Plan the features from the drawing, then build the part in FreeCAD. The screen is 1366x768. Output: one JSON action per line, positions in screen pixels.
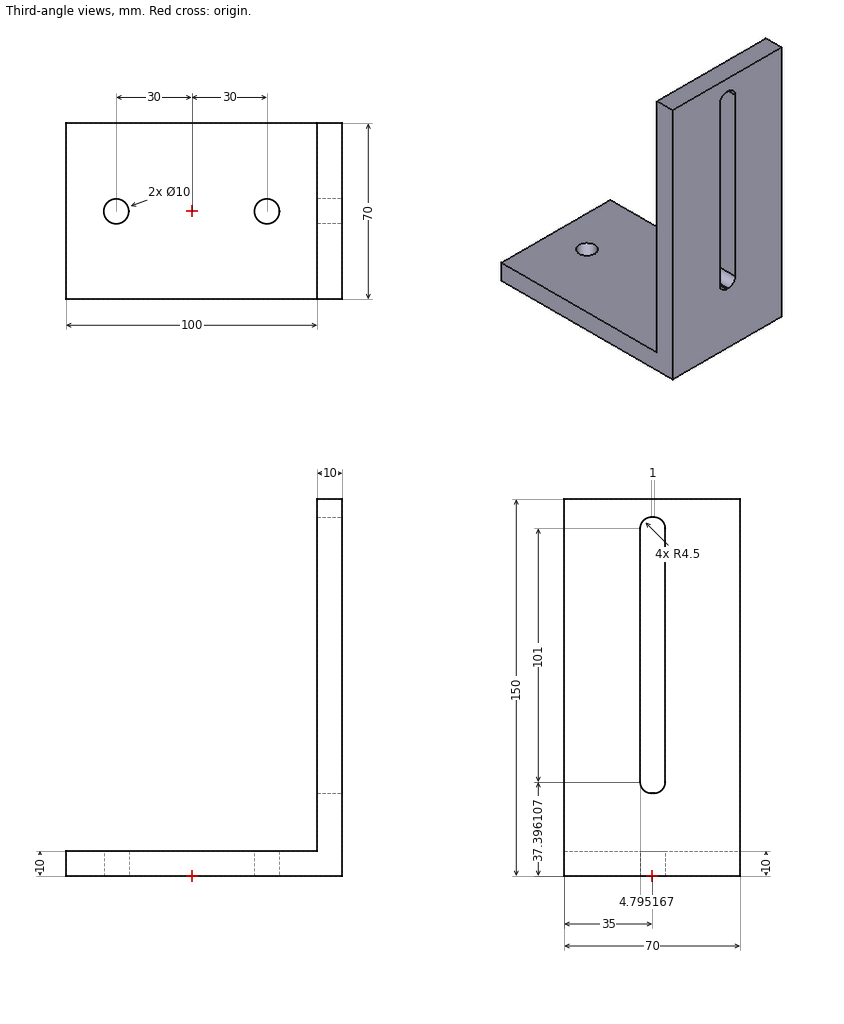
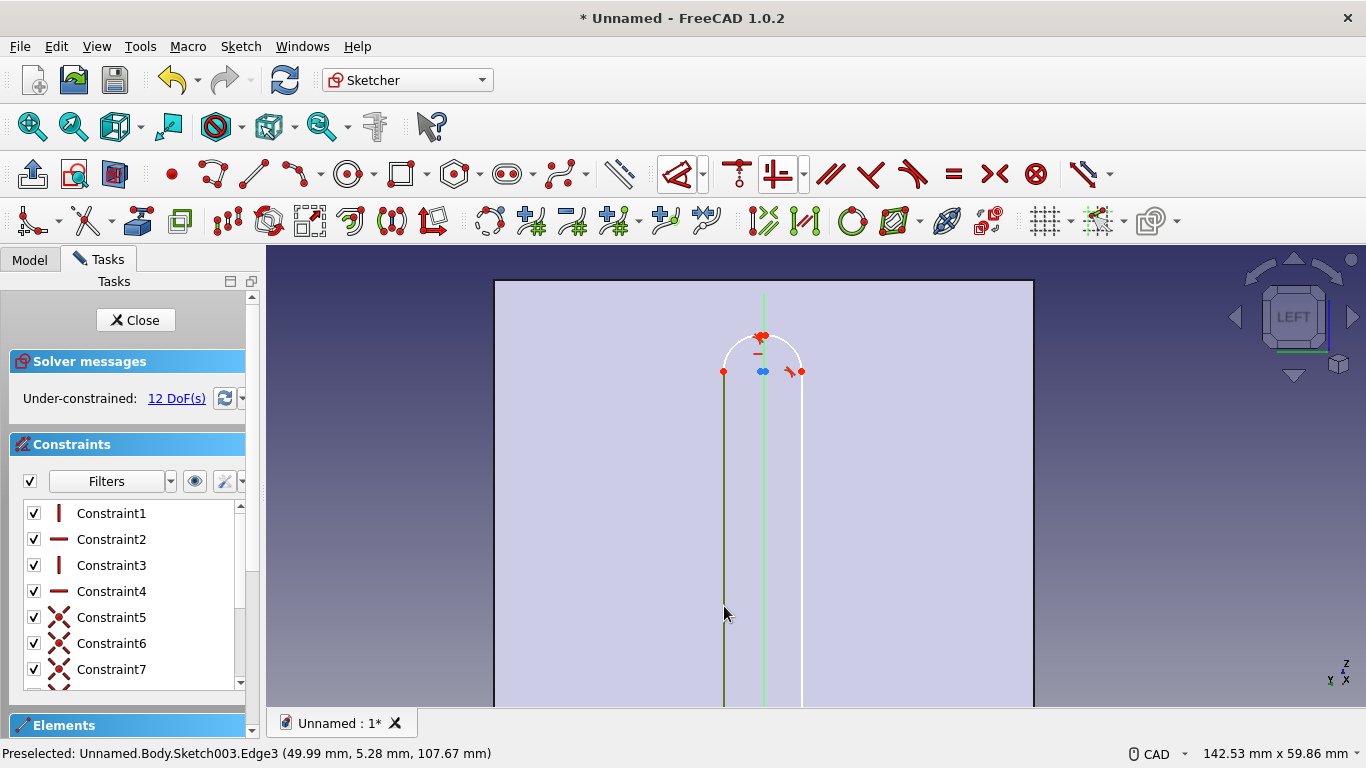
{"action": "left_click", "coordinate": [744, 339]}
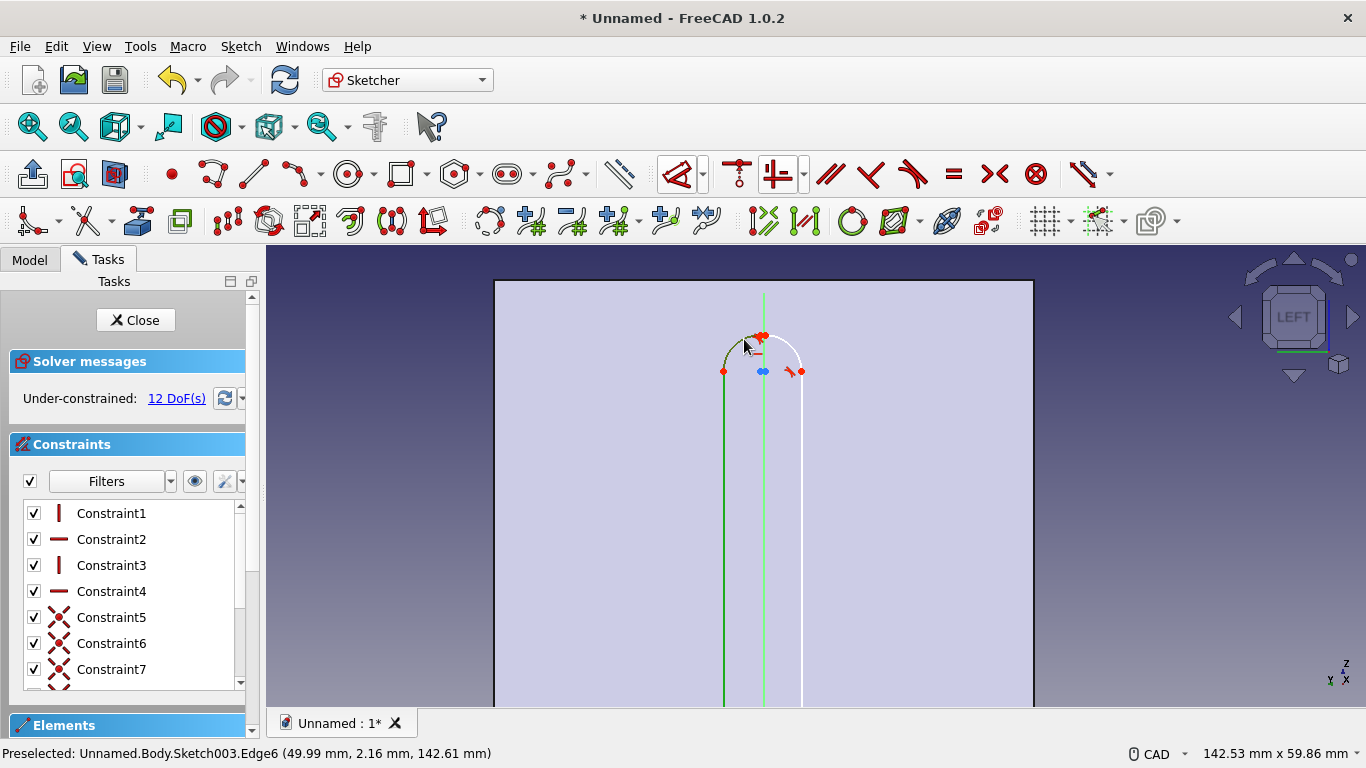
{"action": "left_click", "coordinate": [913, 174]}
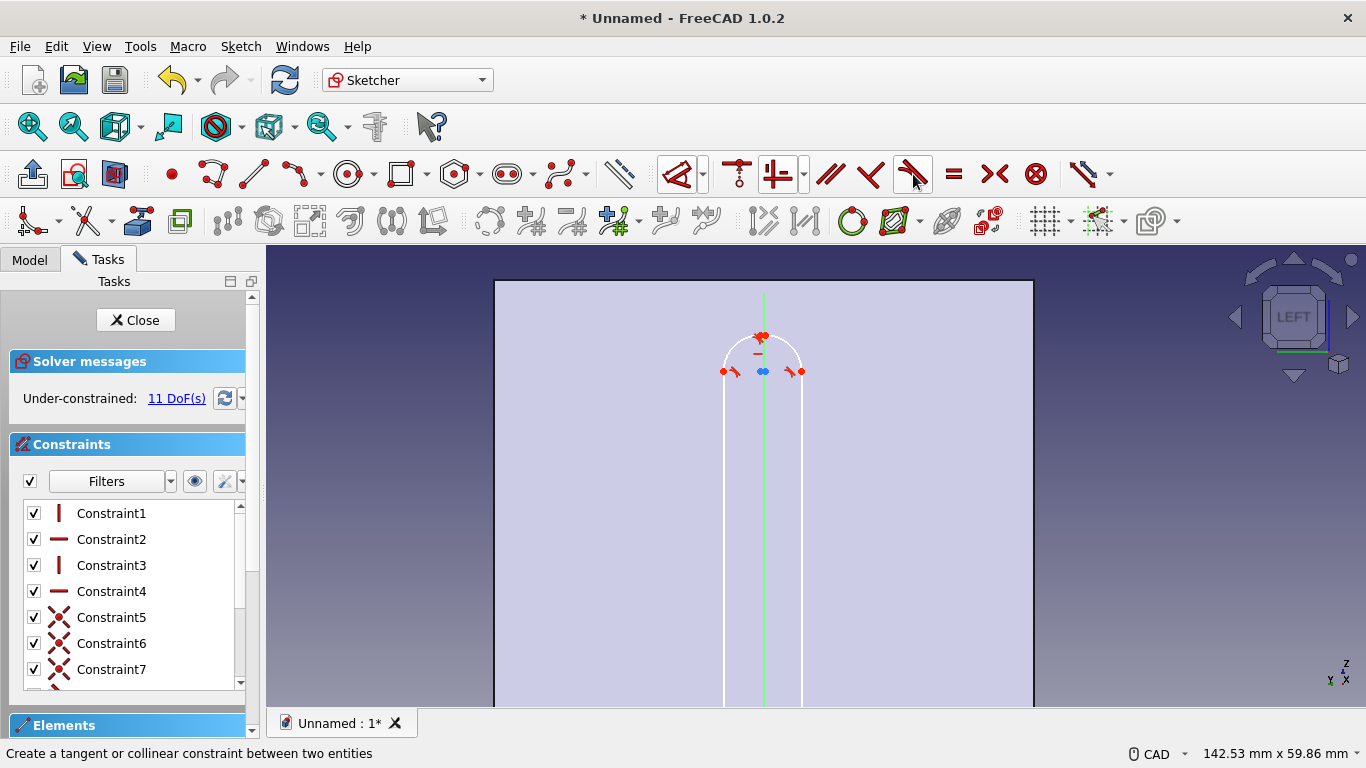
{"action": "left_click", "coordinate": [724, 606]}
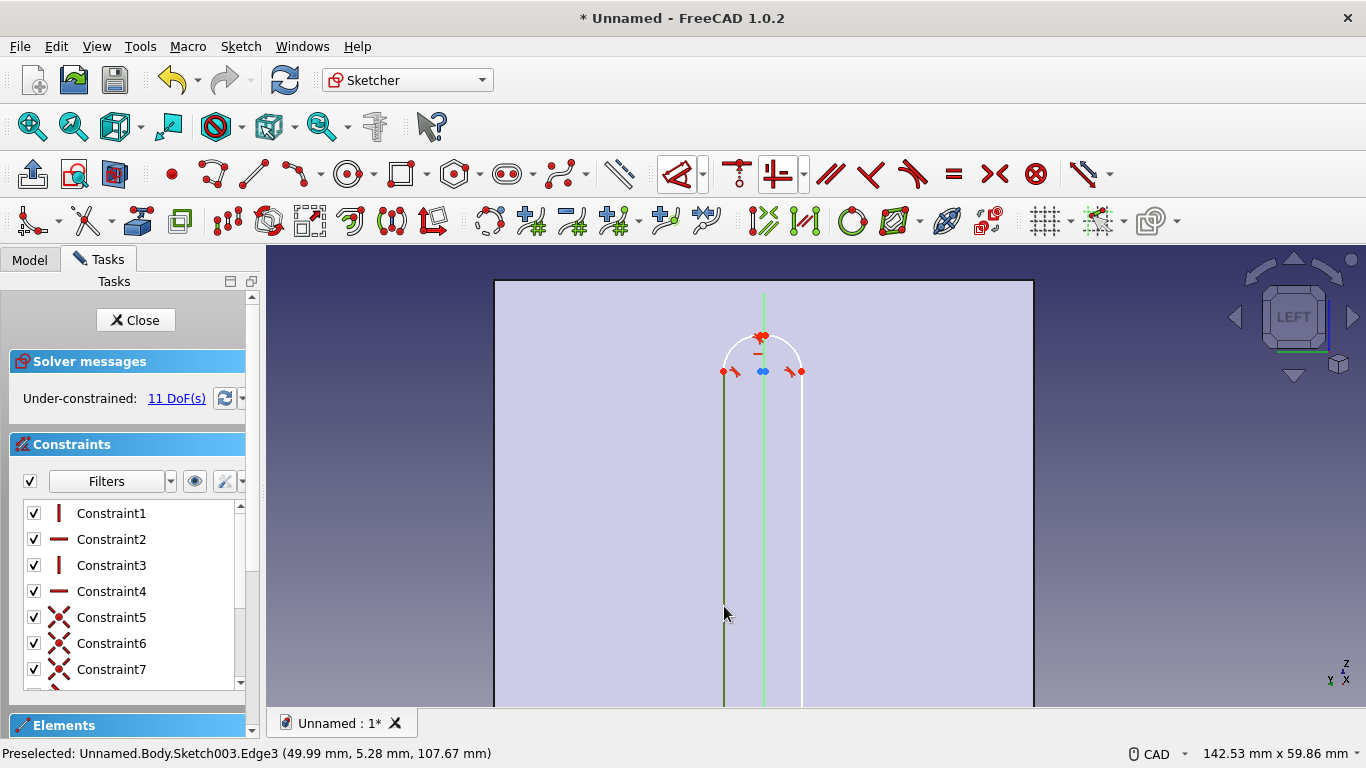
{"action": "scroll", "coordinate": [742, 342], "scroll_direction": "down", "scroll_amount": 7}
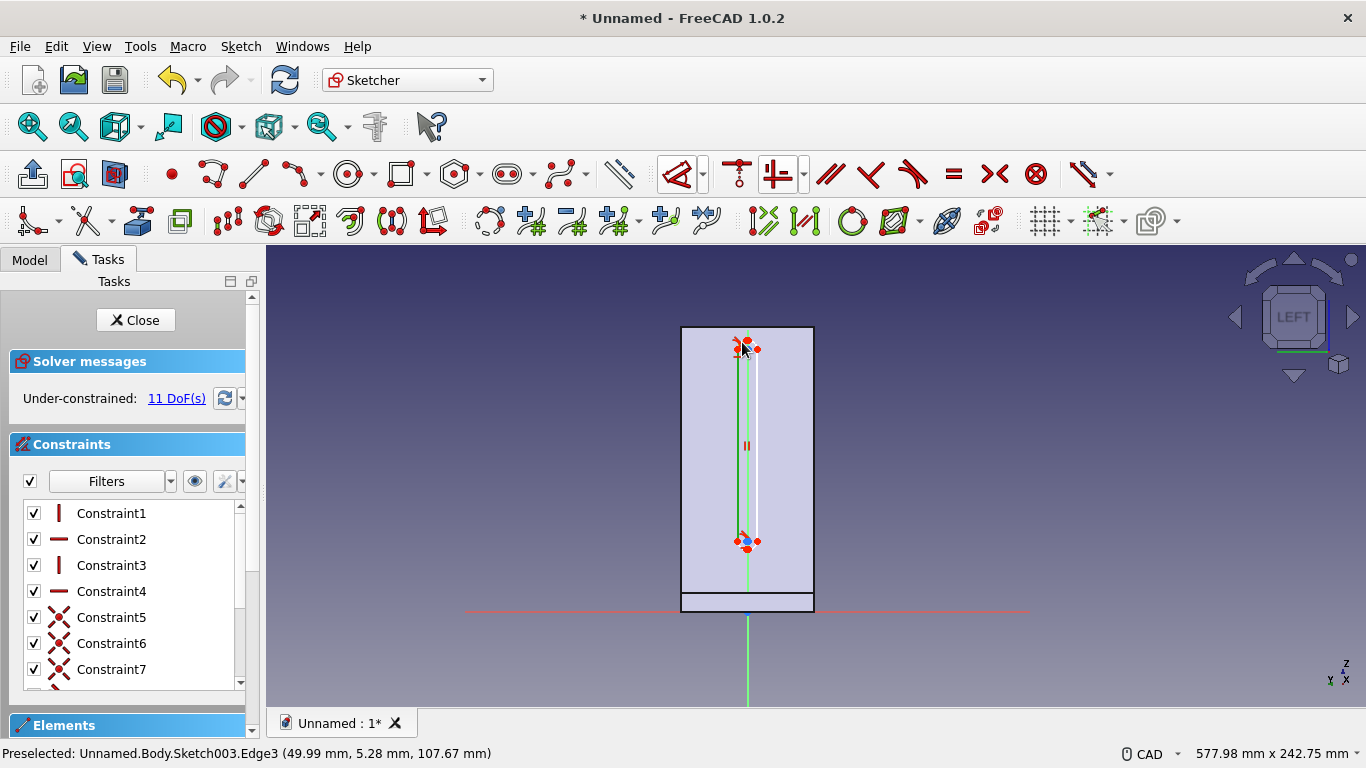
{"action": "scroll", "coordinate": [739, 545], "scroll_direction": "up", "scroll_amount": 7}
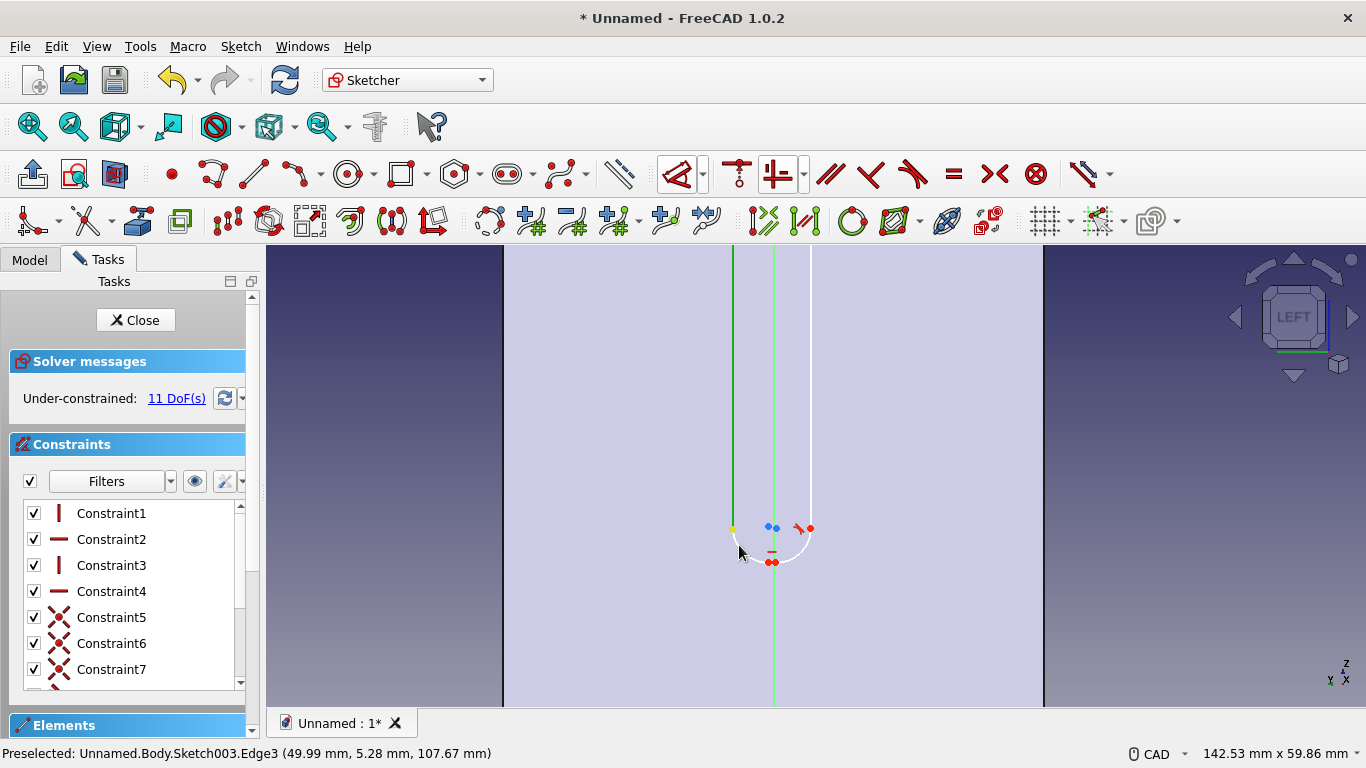
{"action": "left_click", "coordinate": [737, 545]}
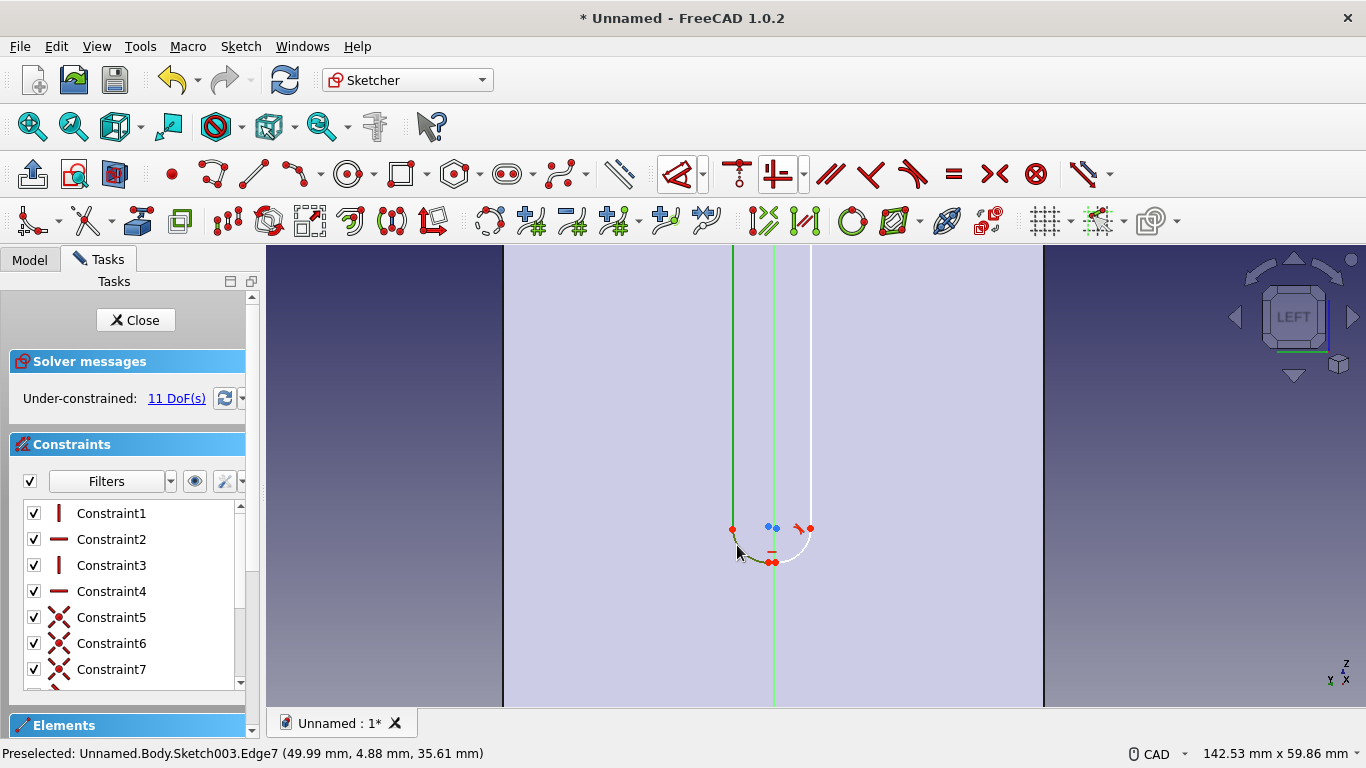
{"action": "left_click", "coordinate": [913, 174]}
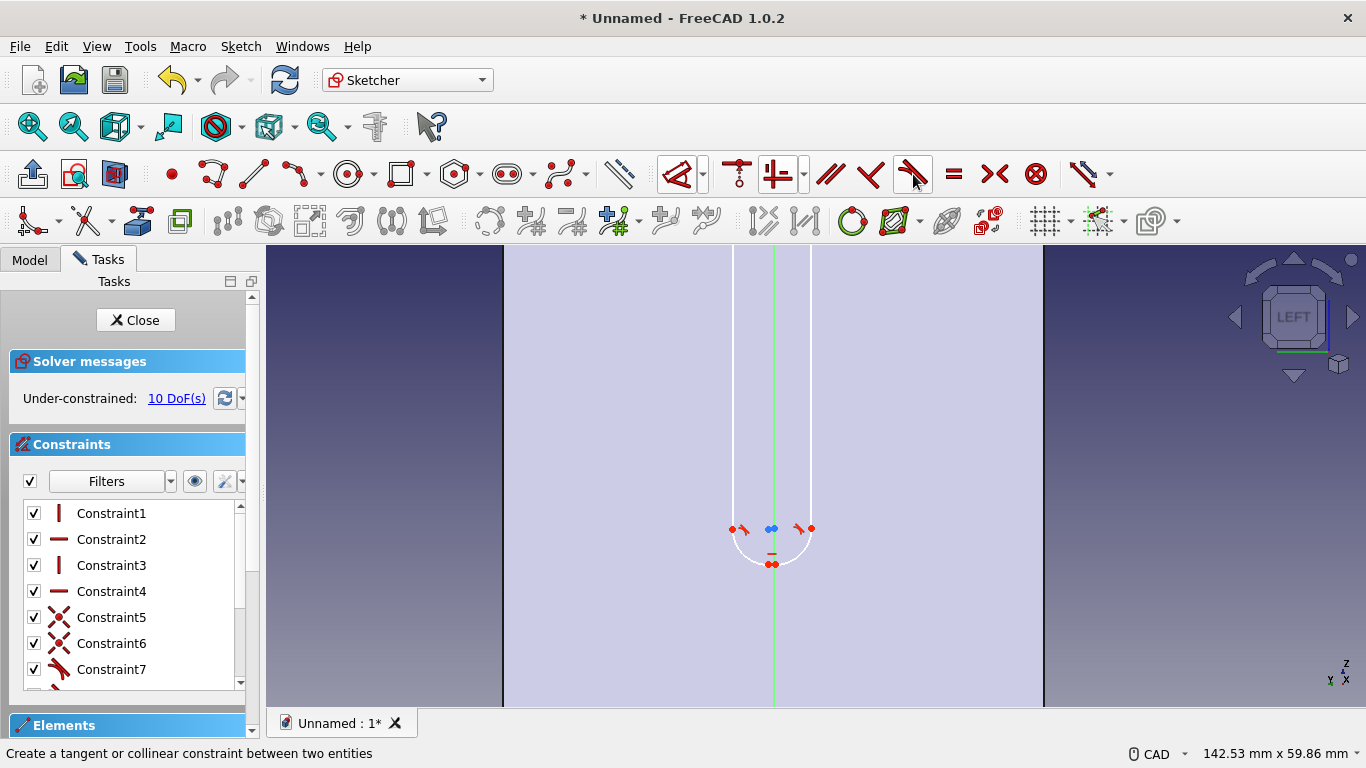
{"action": "scroll", "coordinate": [772, 565], "scroll_direction": "up", "scroll_amount": 7}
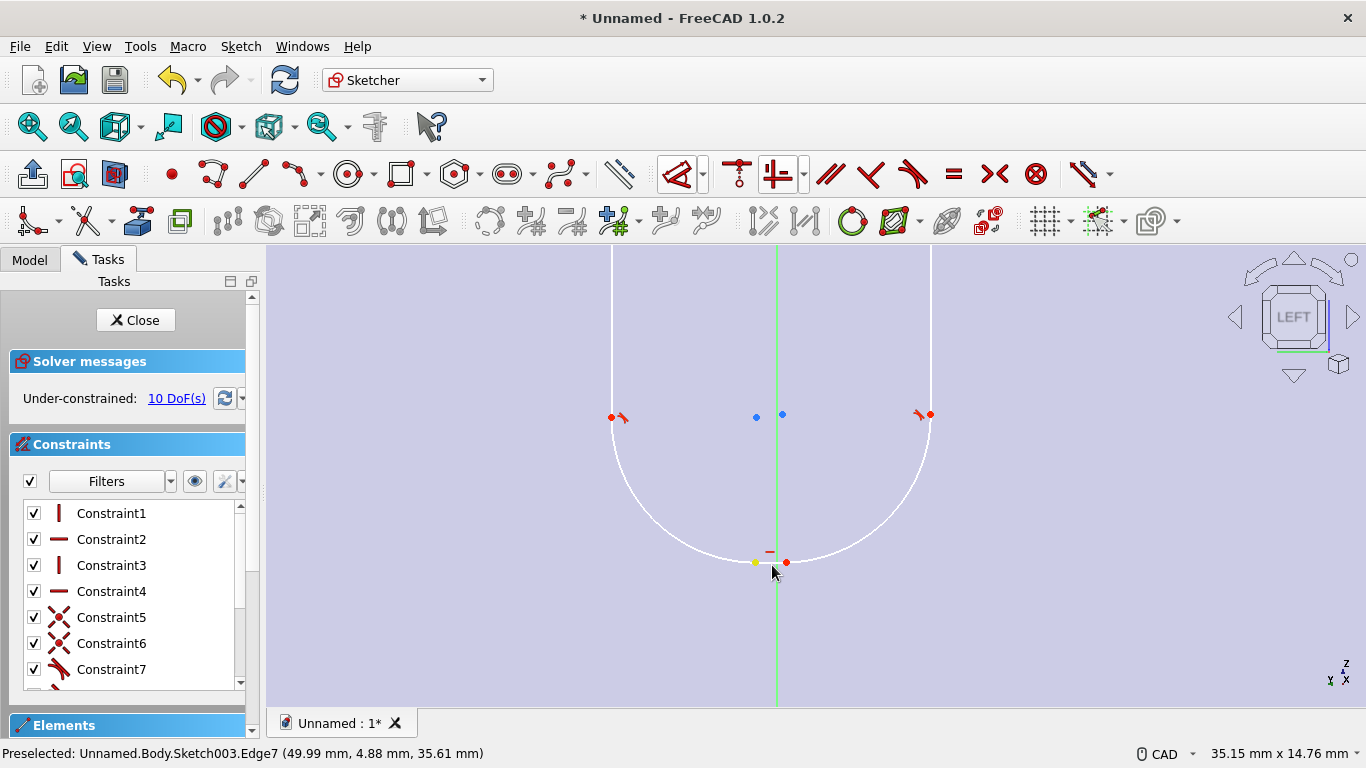
{"action": "left_click", "coordinate": [771, 563]}